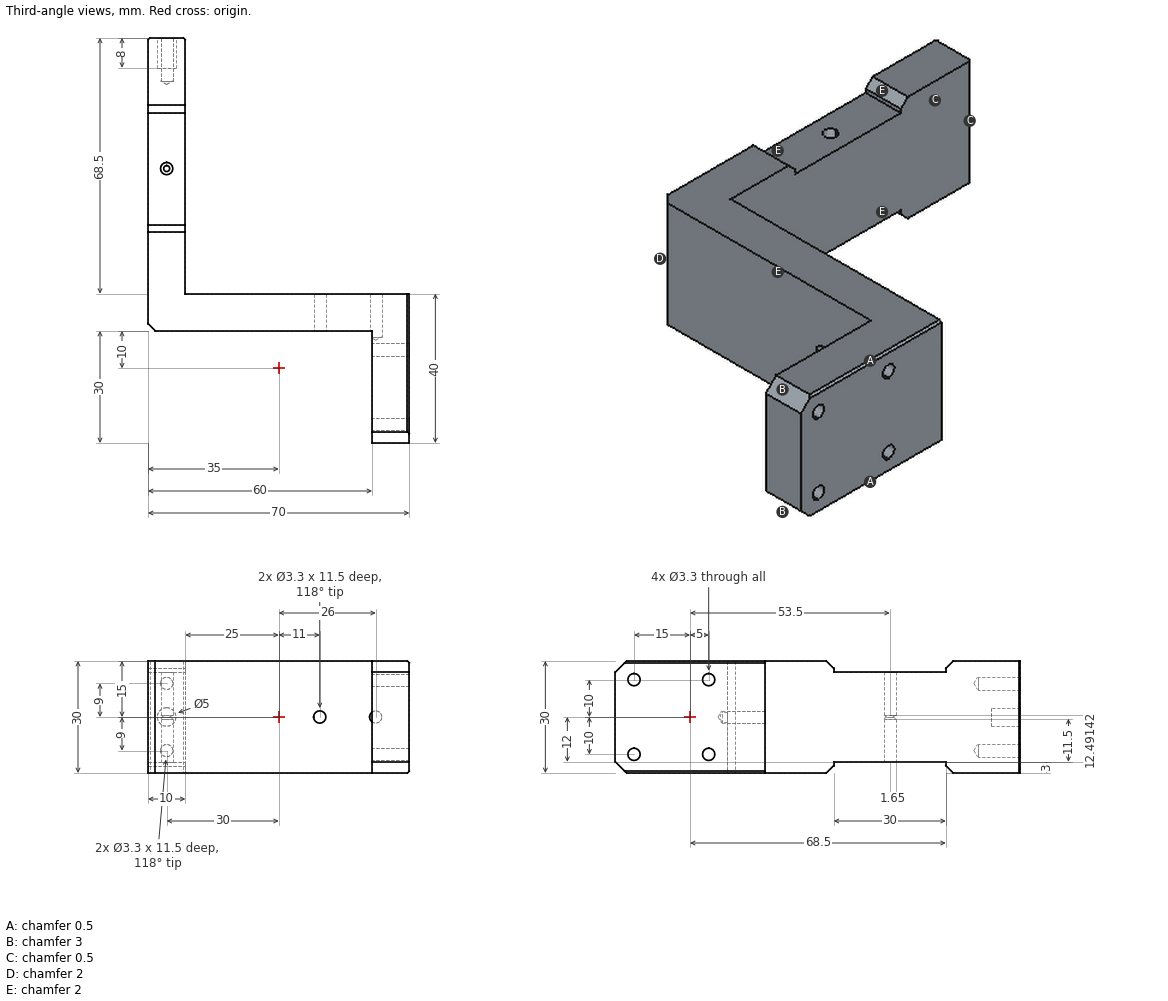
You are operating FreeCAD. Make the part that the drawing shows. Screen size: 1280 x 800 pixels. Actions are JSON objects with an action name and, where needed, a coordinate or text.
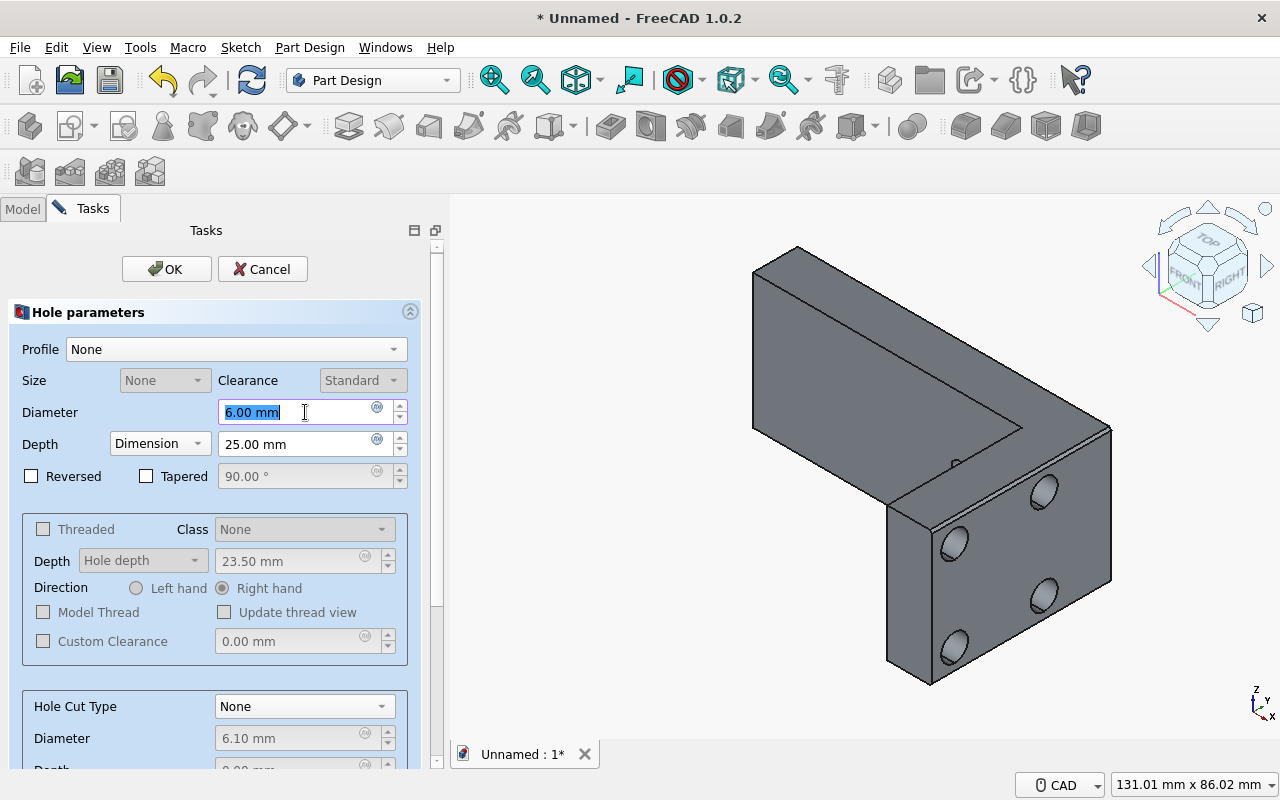
{"action": "type", "text": "3.3"}
{"action": "key", "text": "Tab"}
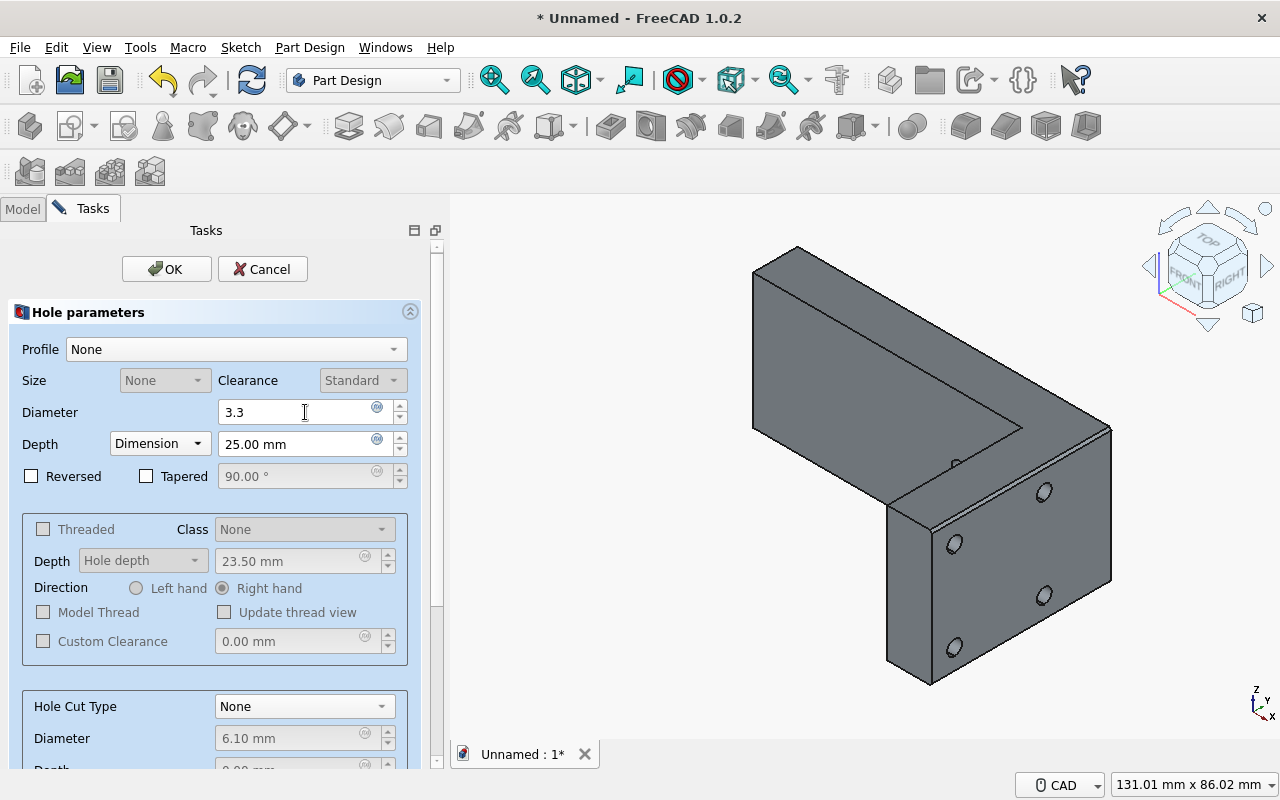
{"action": "left_click", "coordinate": [161, 444]}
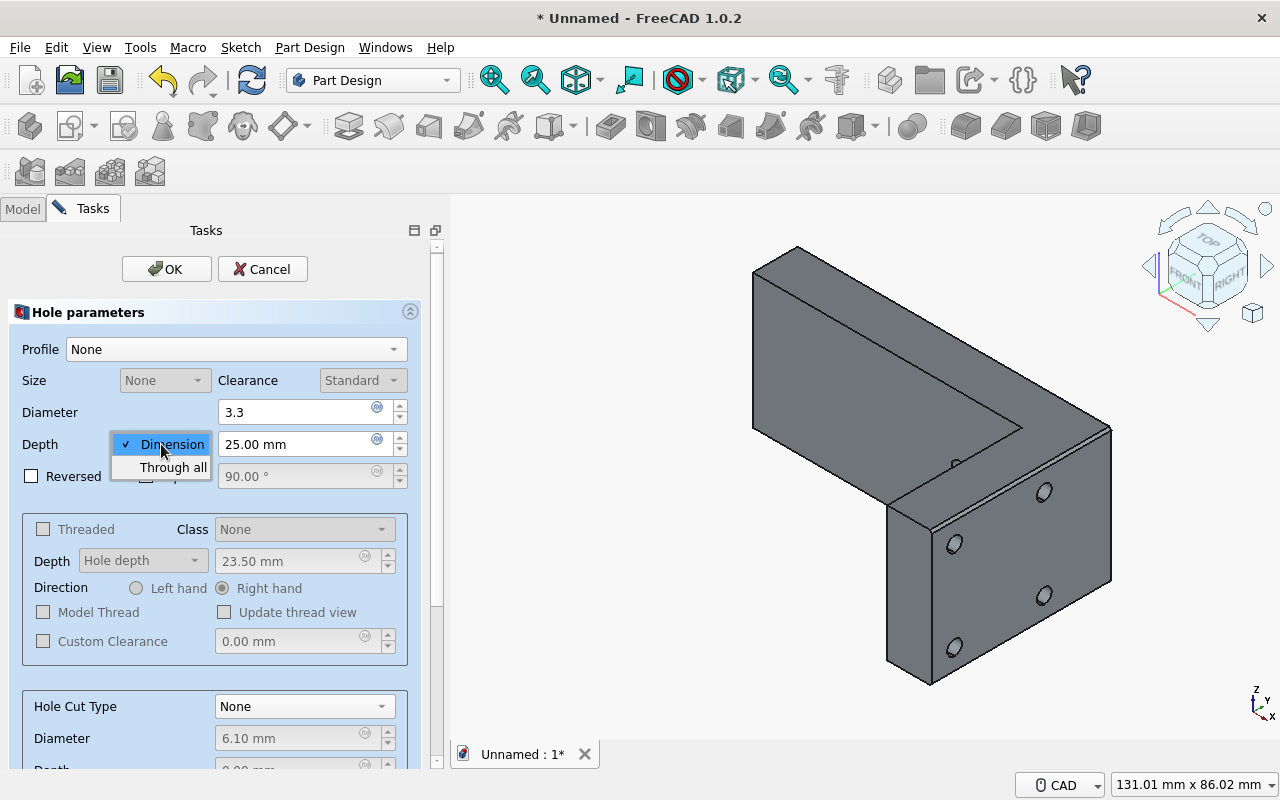
{"action": "left_click", "coordinate": [160, 468]}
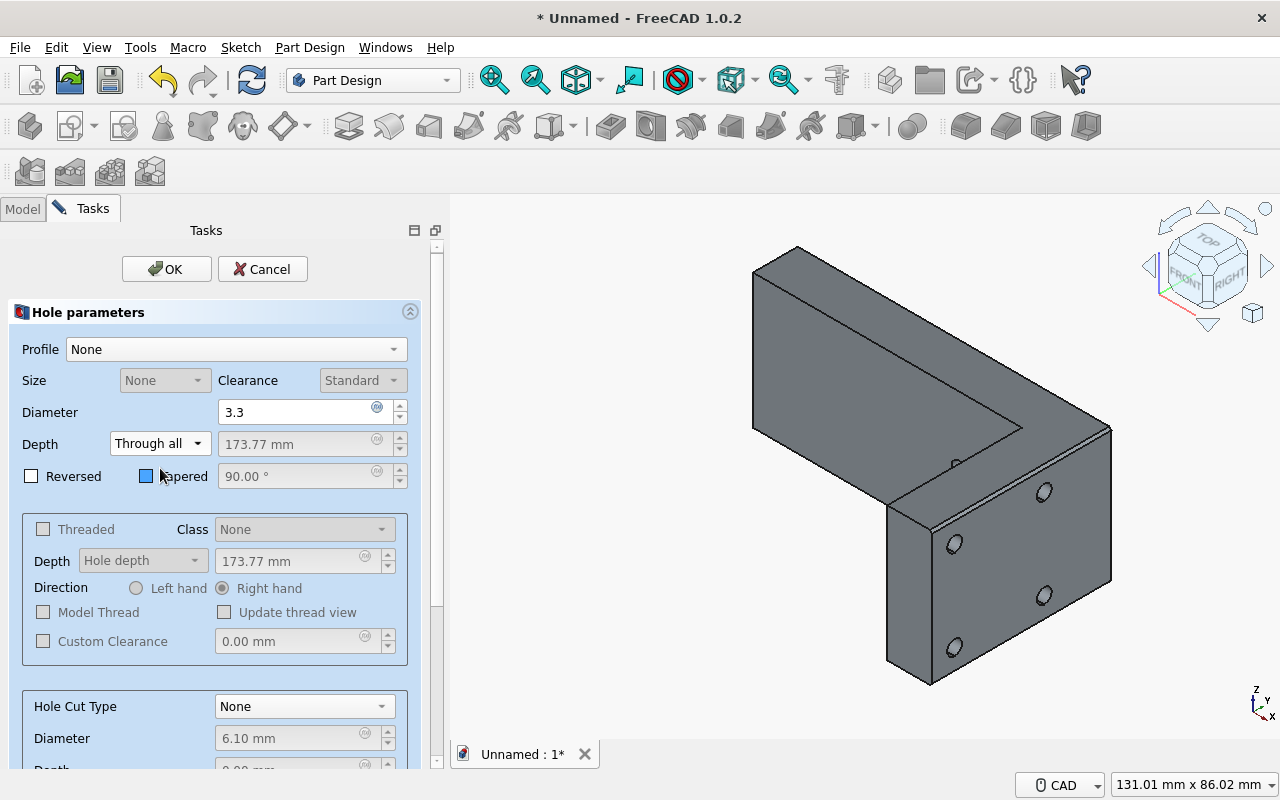
{"action": "left_click", "coordinate": [167, 269]}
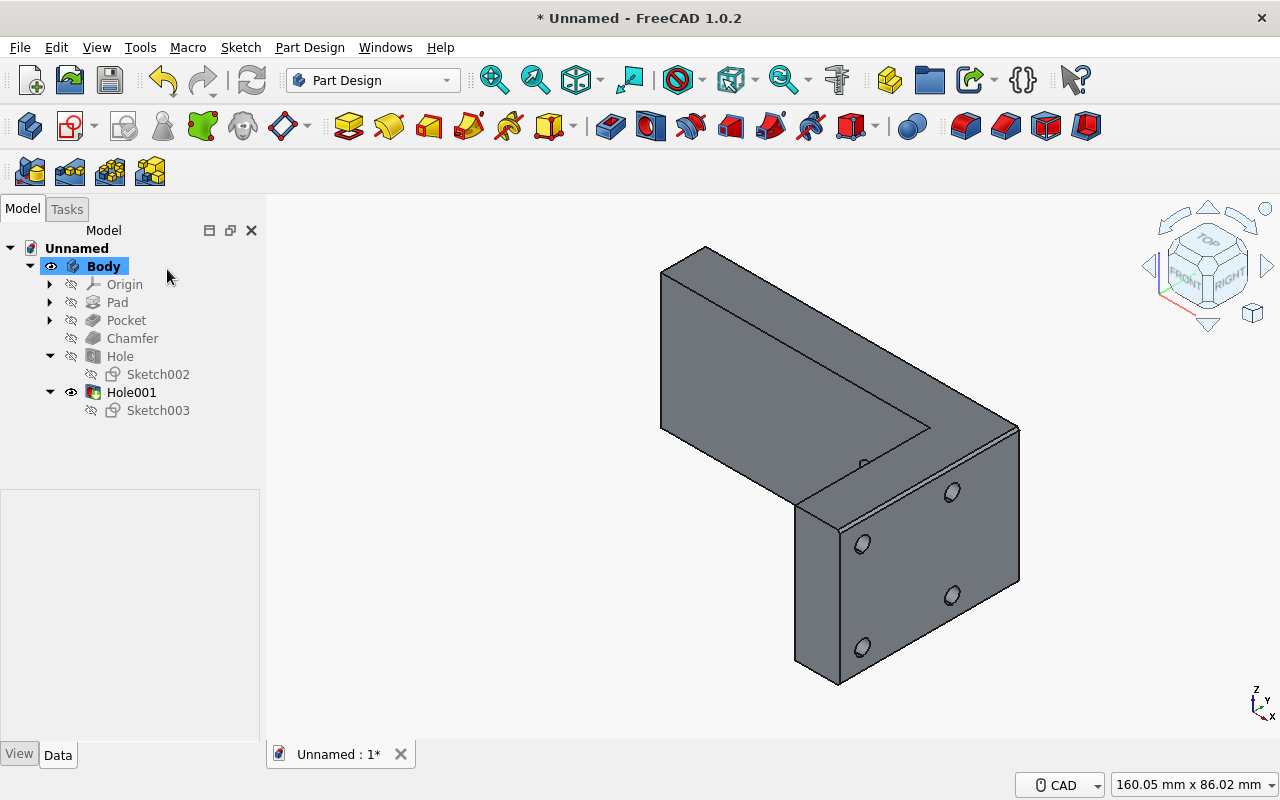
{"action": "left_click", "coordinate": [817, 517]}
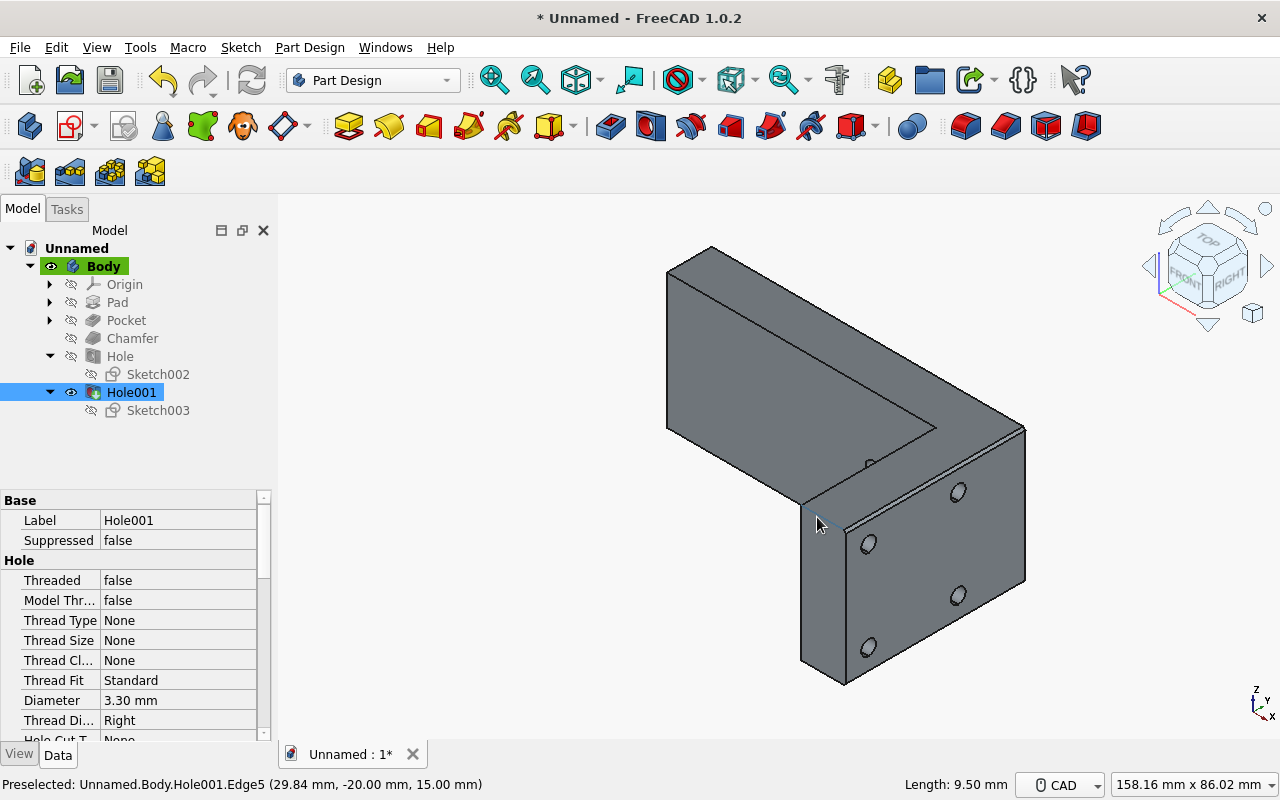
{"action": "key", "text": "2"}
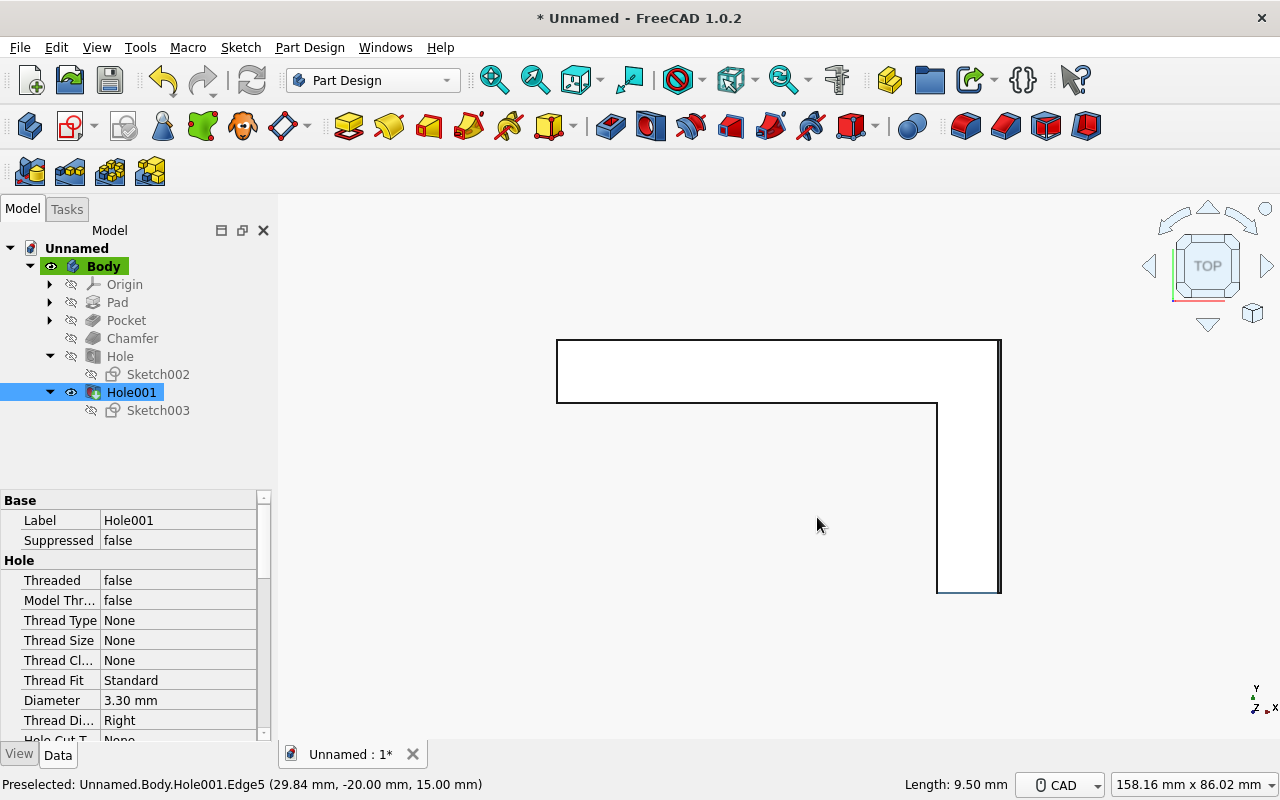
{"action": "key", "text": "0"}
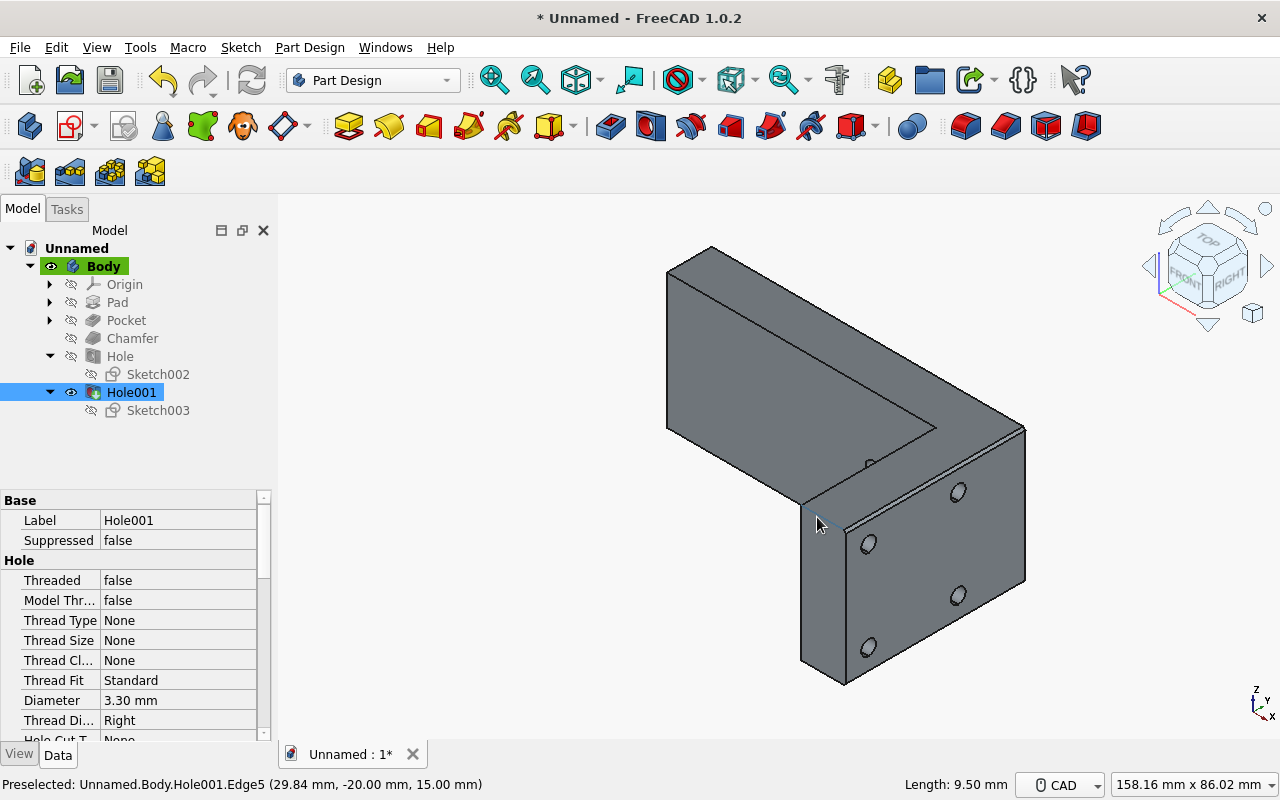
{"action": "key", "text": "1"}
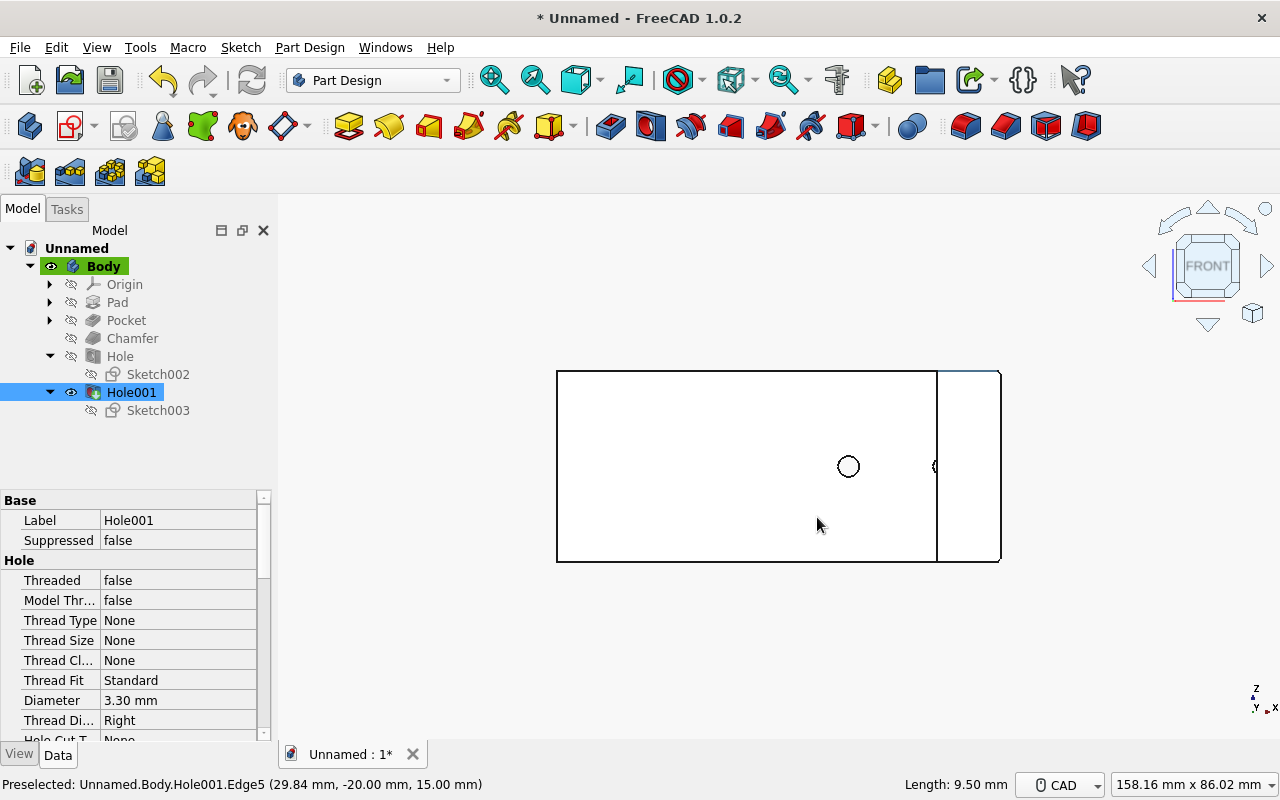
{"action": "key", "text": "v f"}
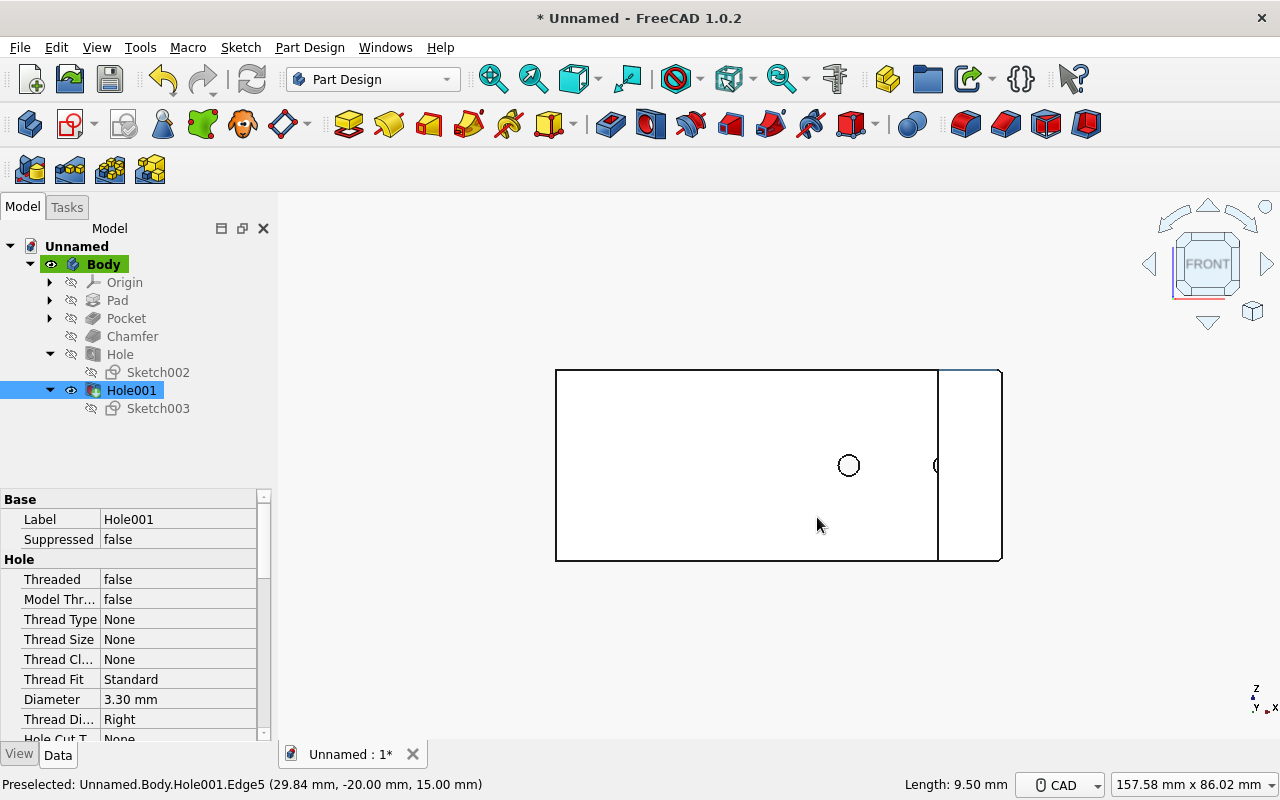
{"action": "left_click", "coordinate": [968, 560], "text": "ctrl"}